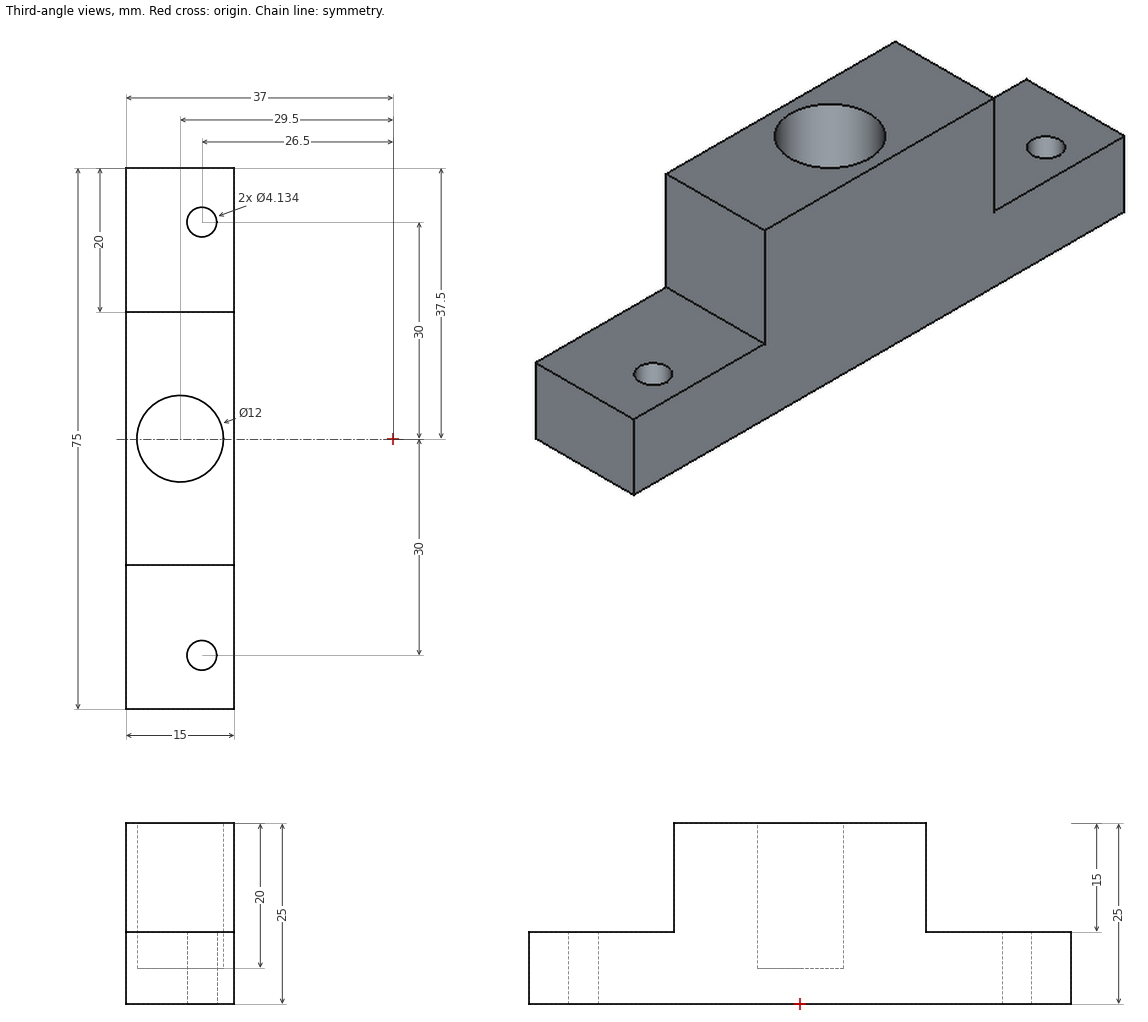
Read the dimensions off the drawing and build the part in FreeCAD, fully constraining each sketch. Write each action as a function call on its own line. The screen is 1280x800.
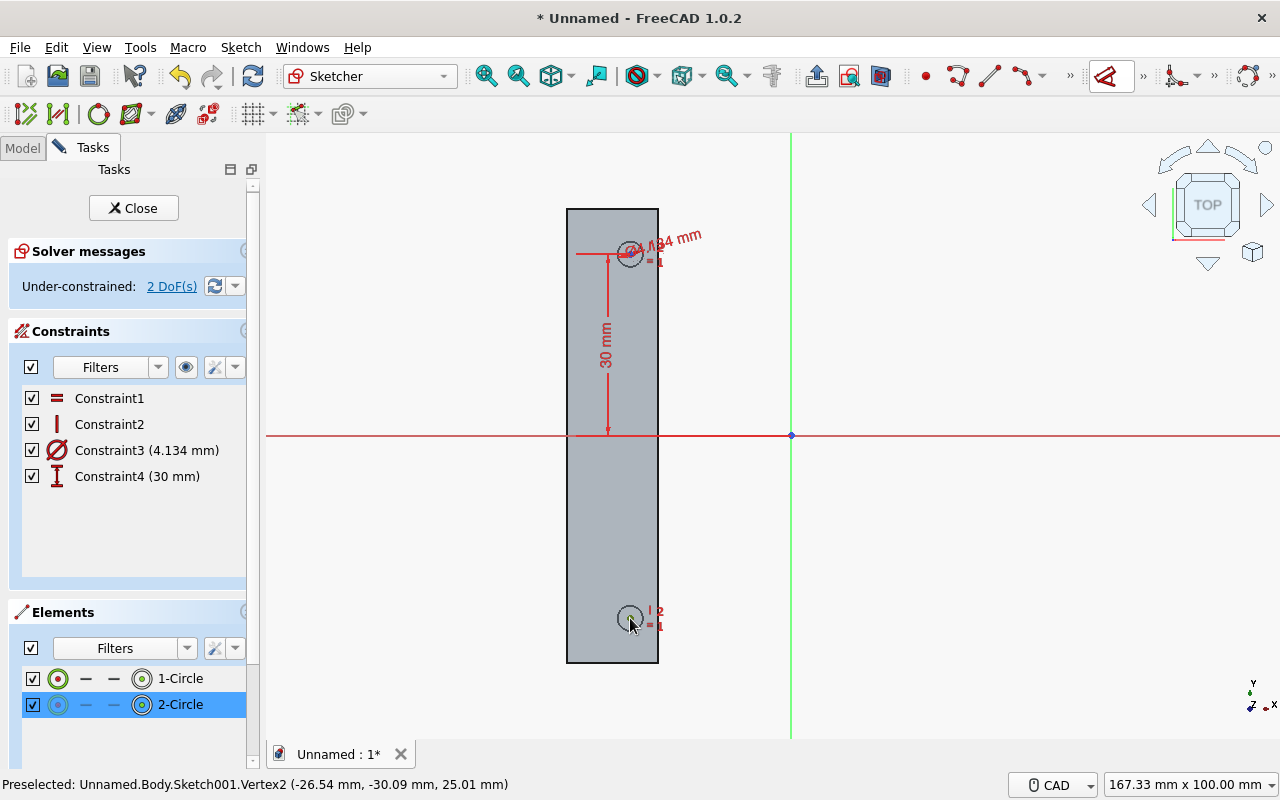
key(i)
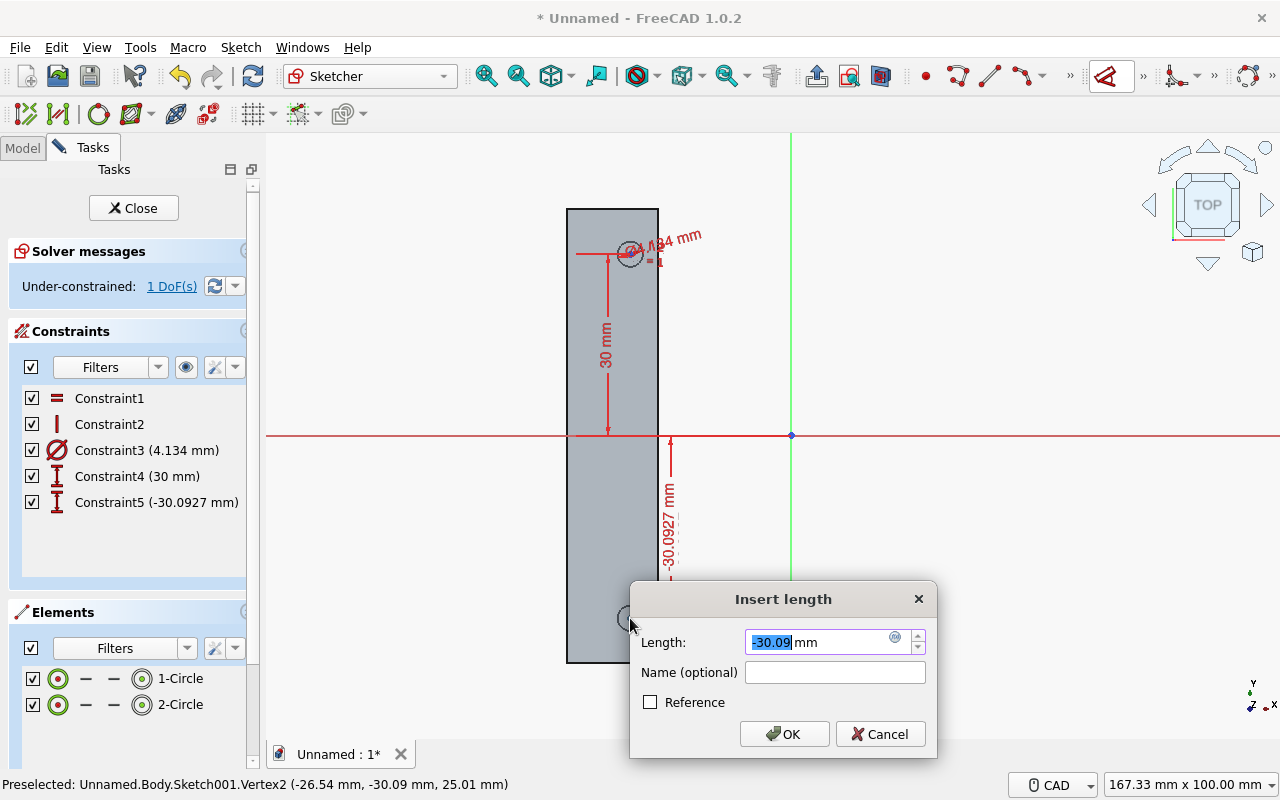
text(-30)
key(Return)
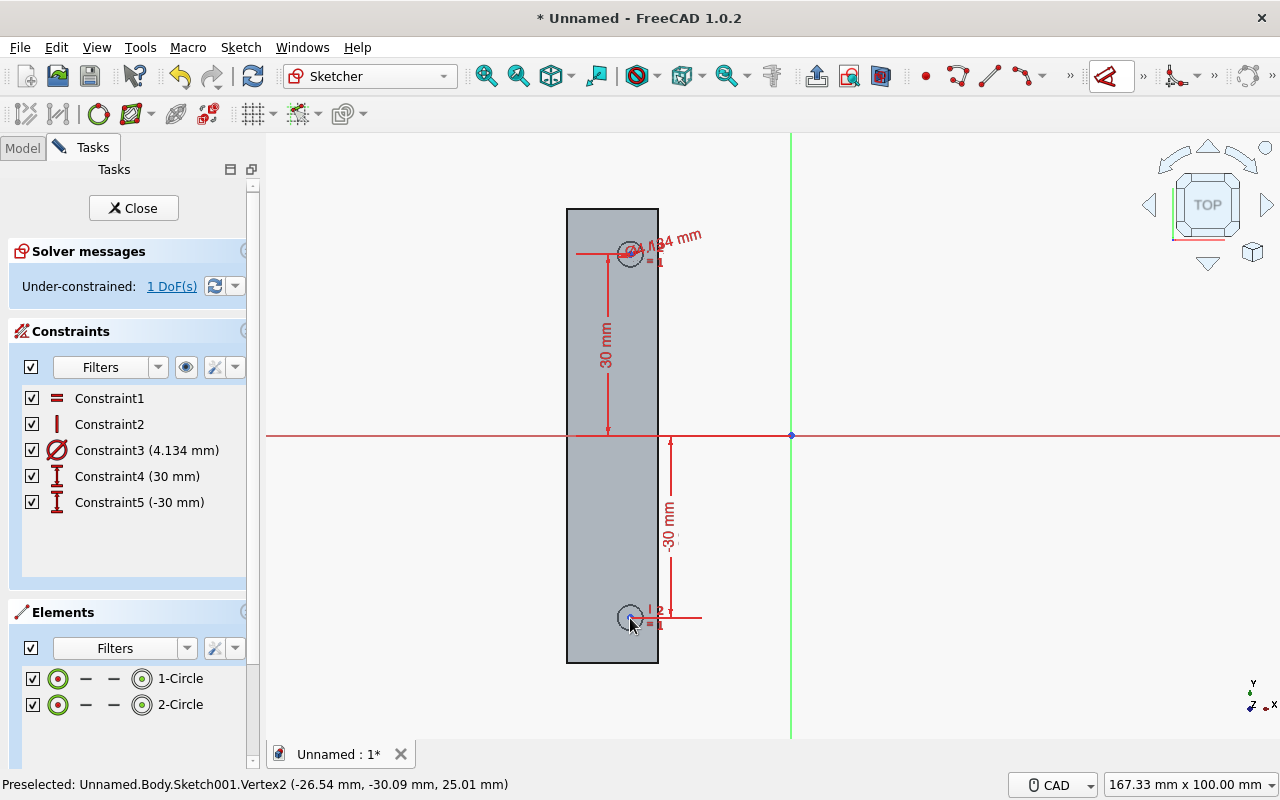
click(630, 254)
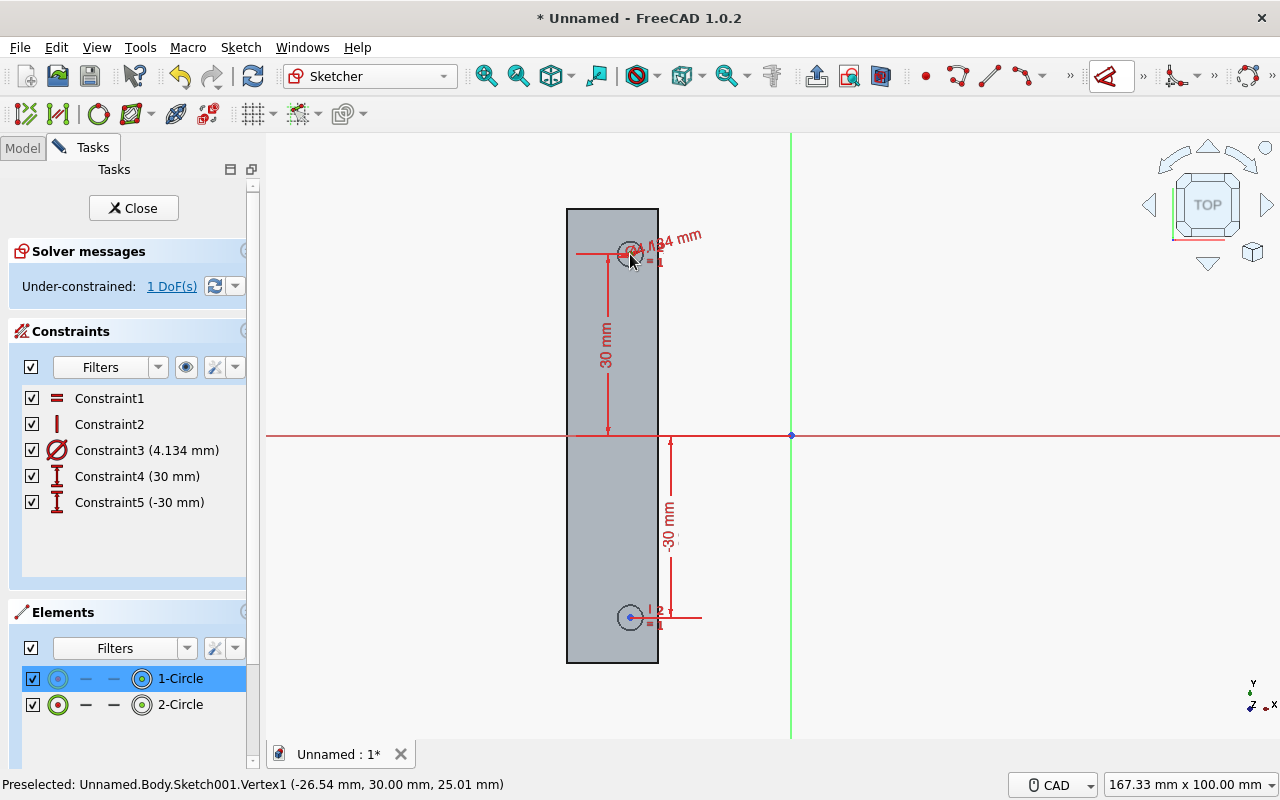
click(1128, 76)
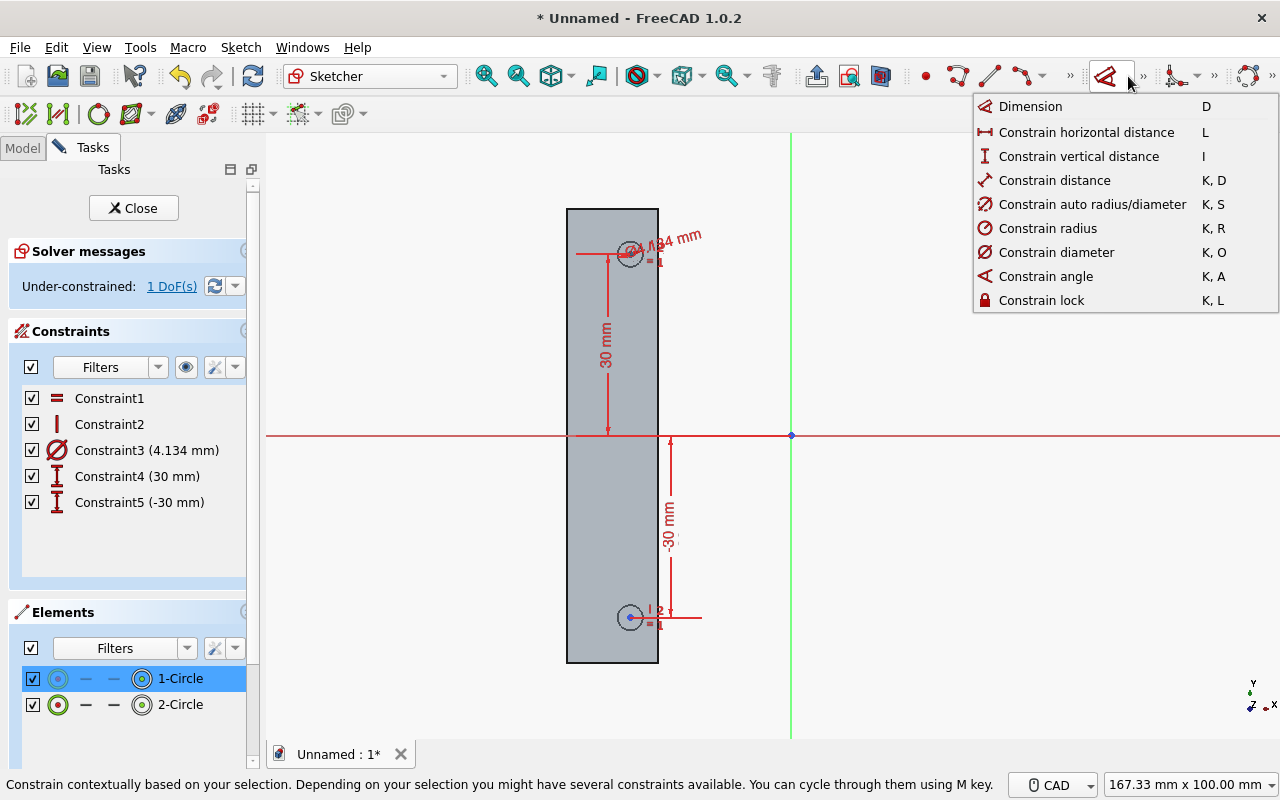
click(1126, 132)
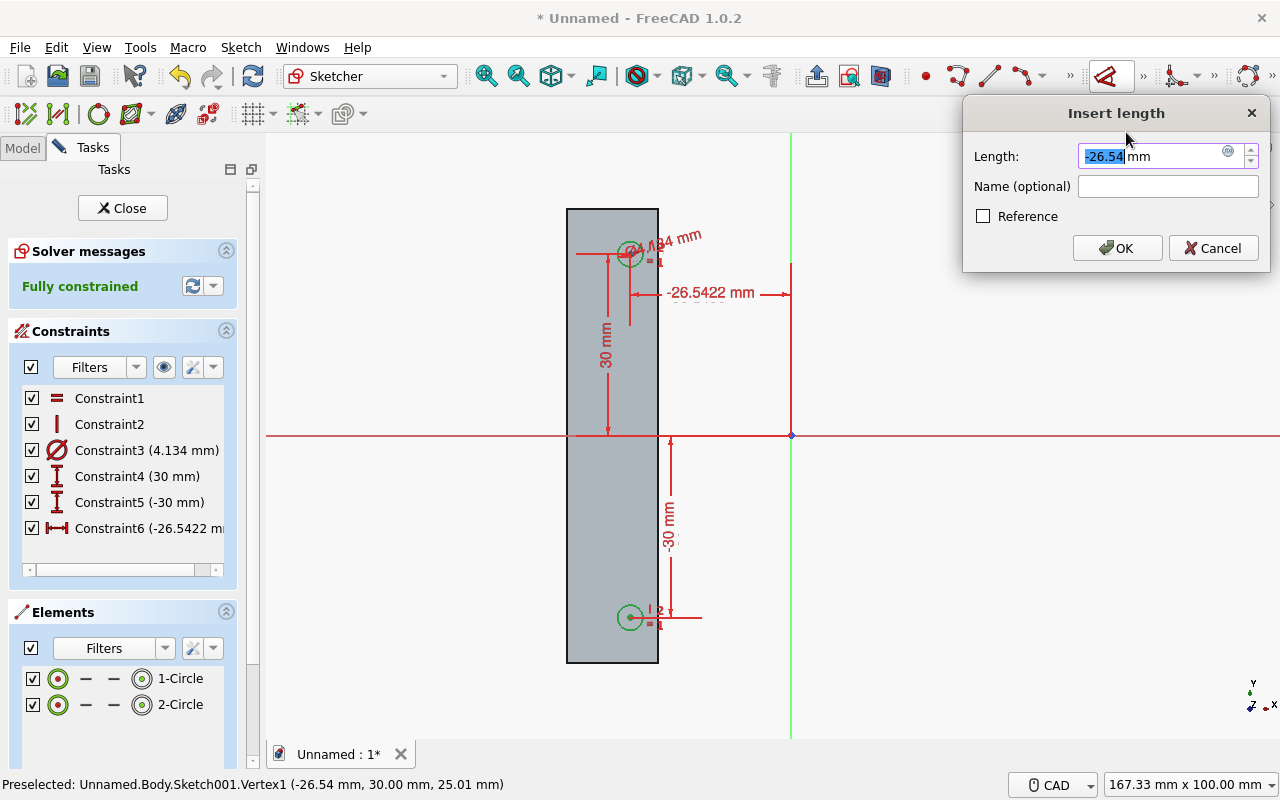
text(-26.5)
key(Return)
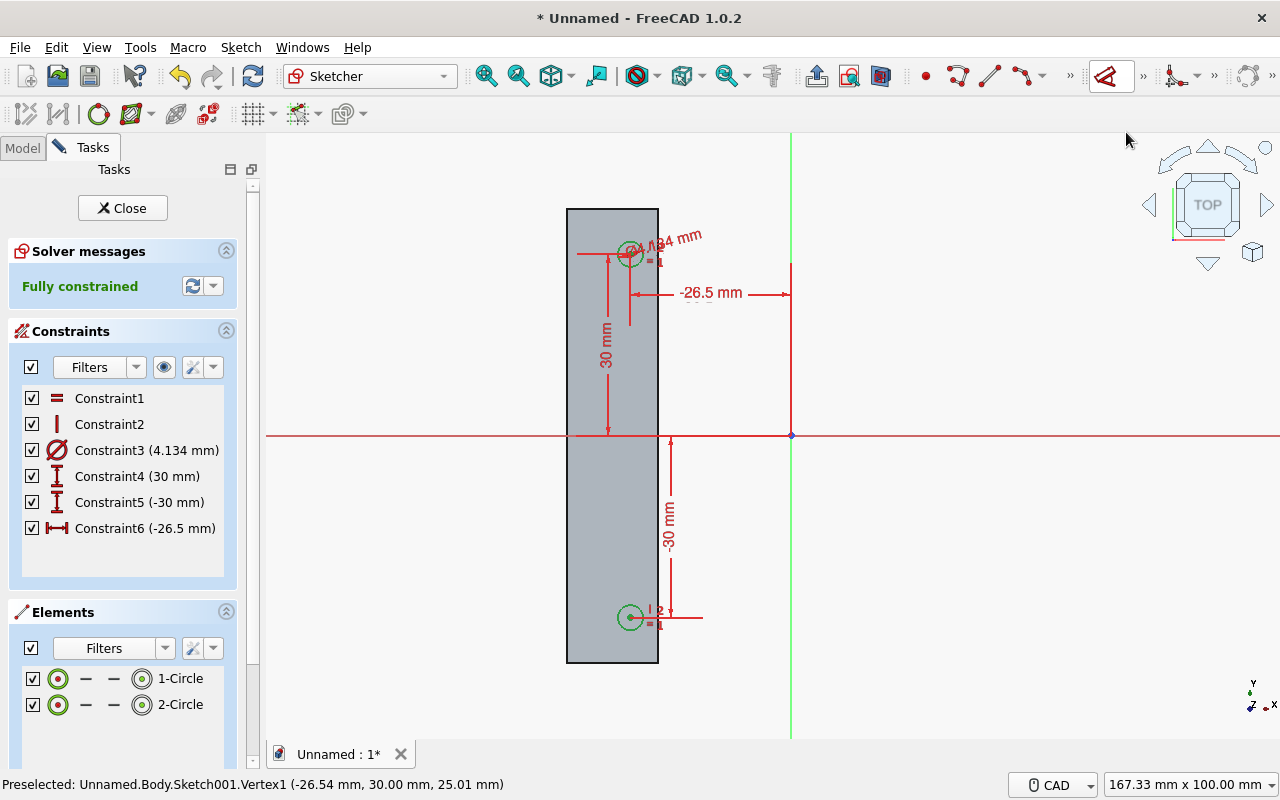
click(123, 208)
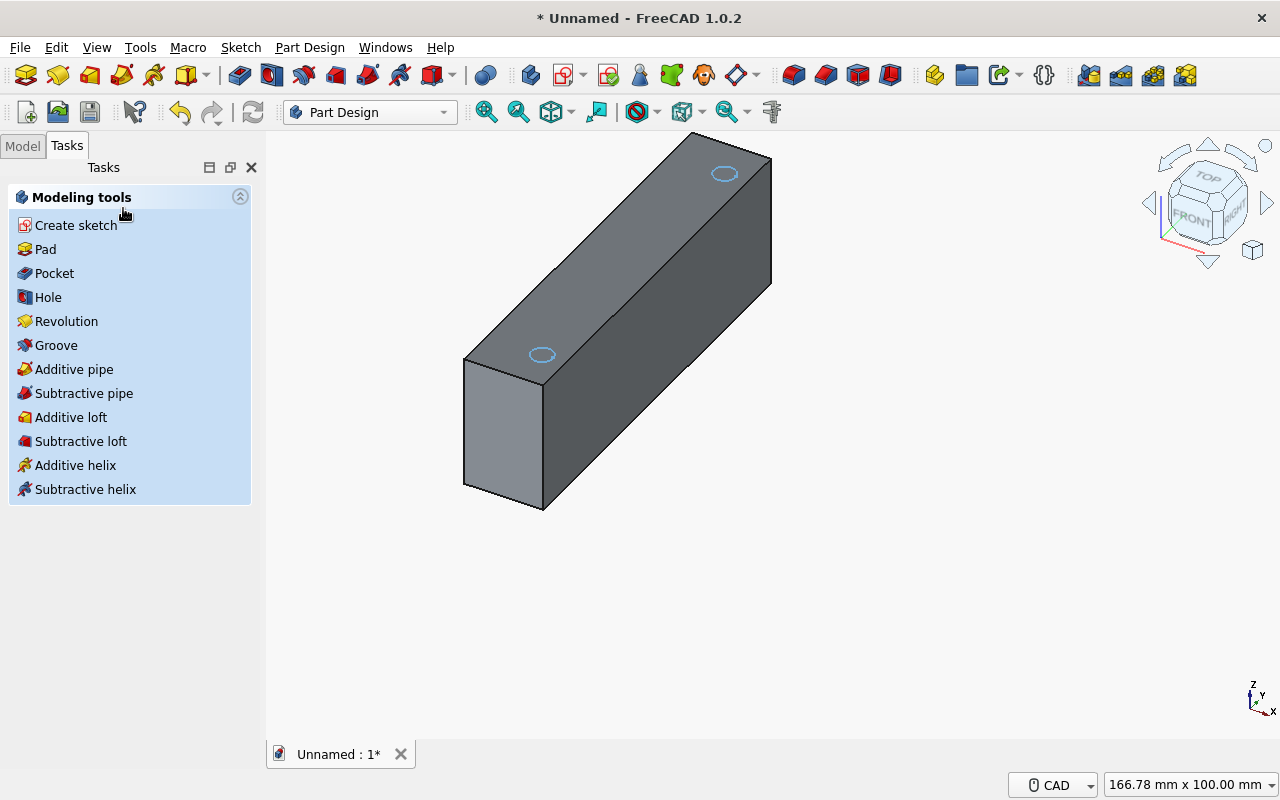
click(240, 76)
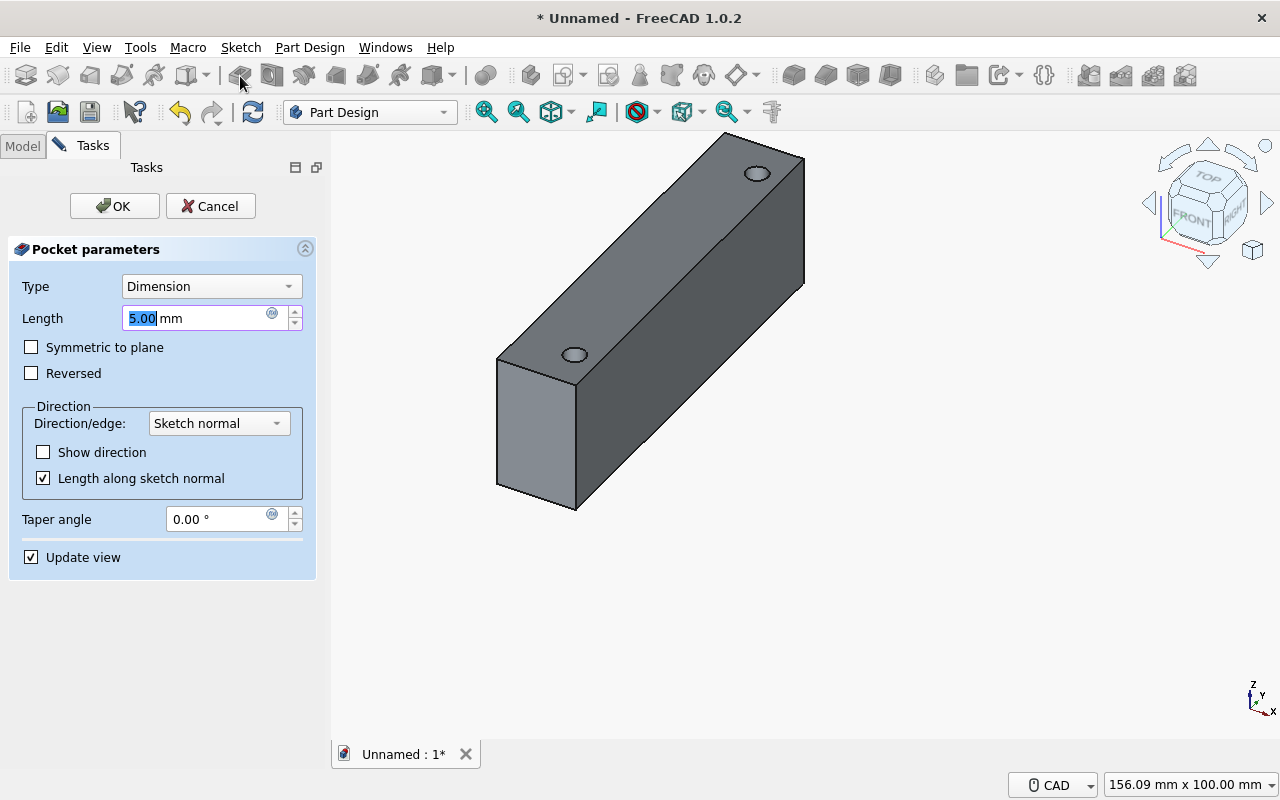
text(25)
key(Tab)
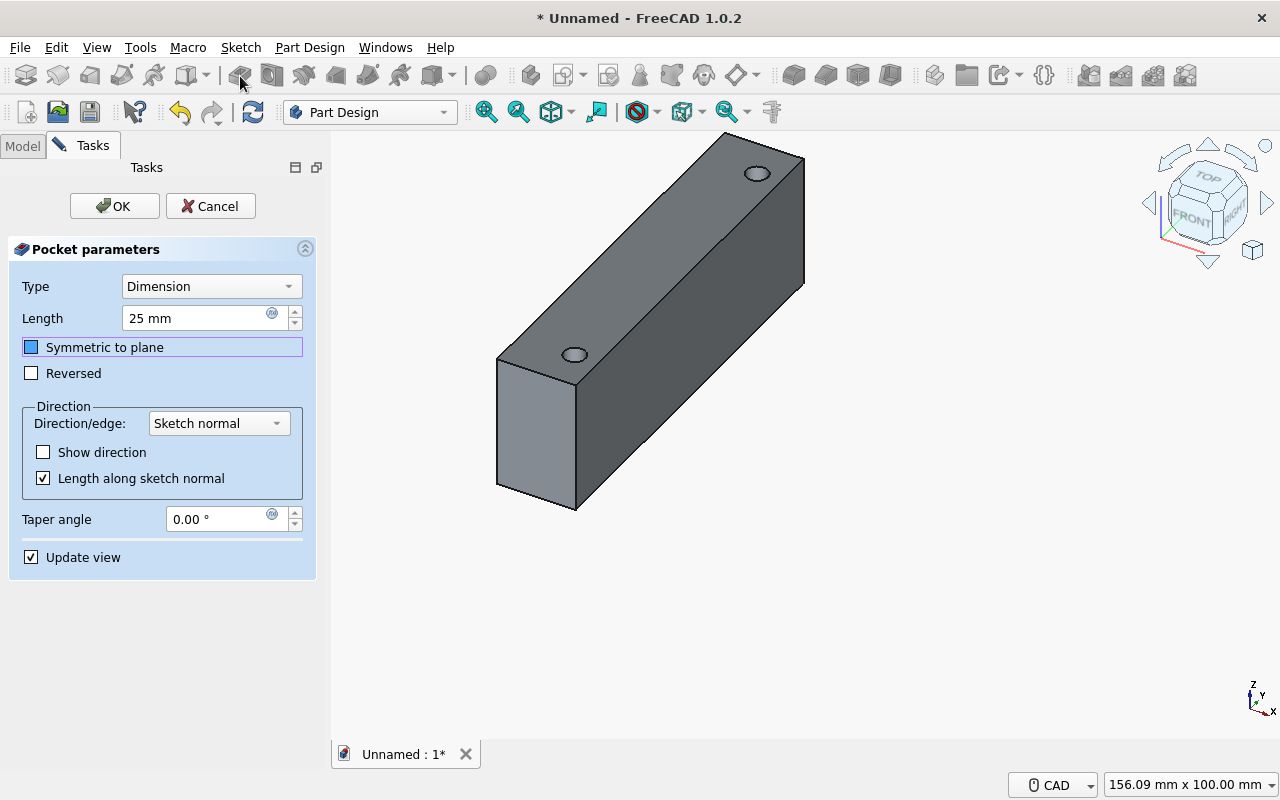
click(115, 206)